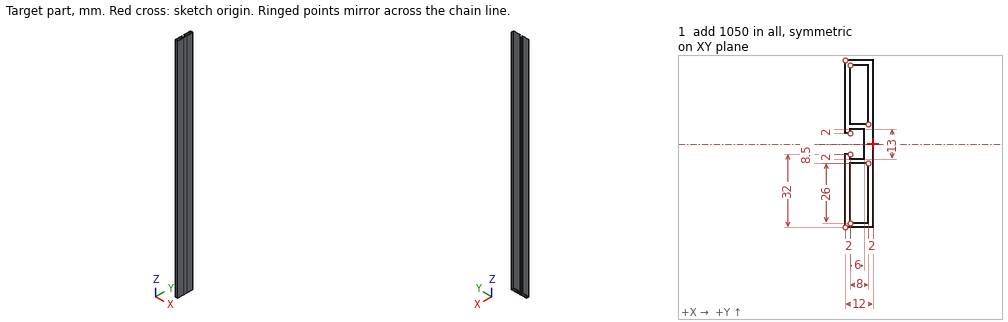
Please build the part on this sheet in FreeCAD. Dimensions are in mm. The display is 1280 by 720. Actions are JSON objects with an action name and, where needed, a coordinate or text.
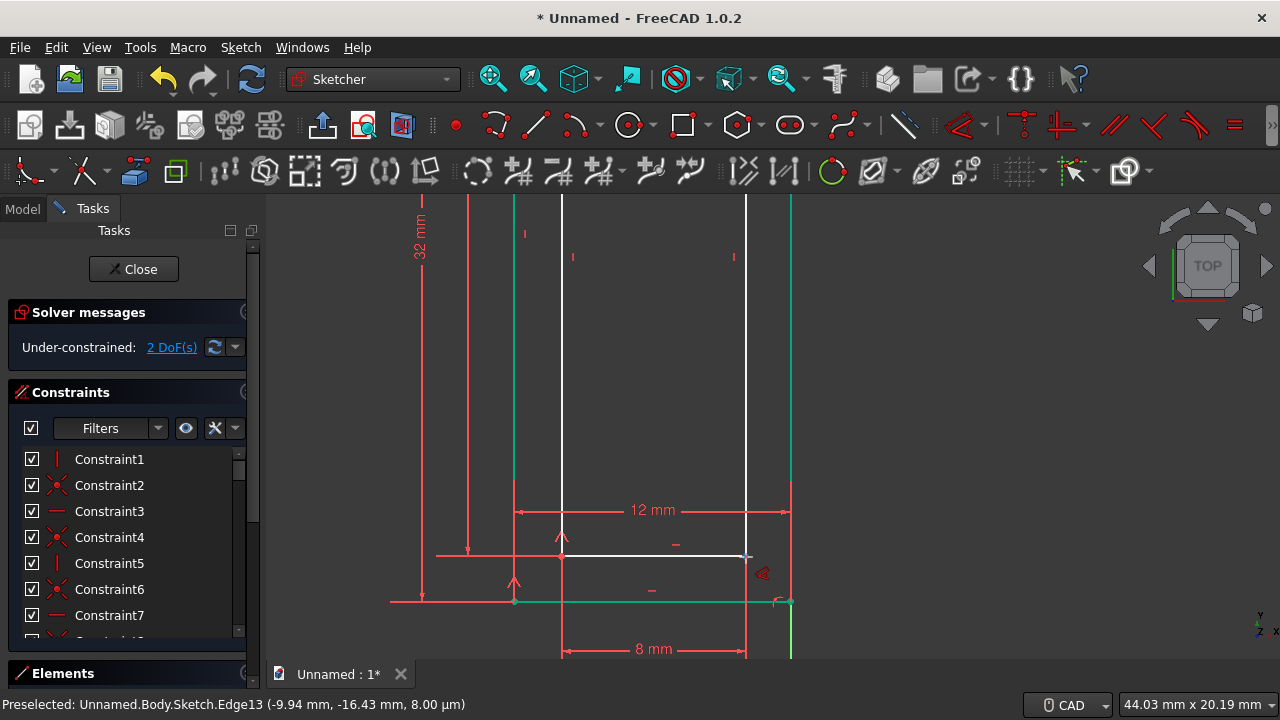
{"action": "left_click", "coordinate": [746, 556]}
{"action": "left_click", "coordinate": [768, 590]}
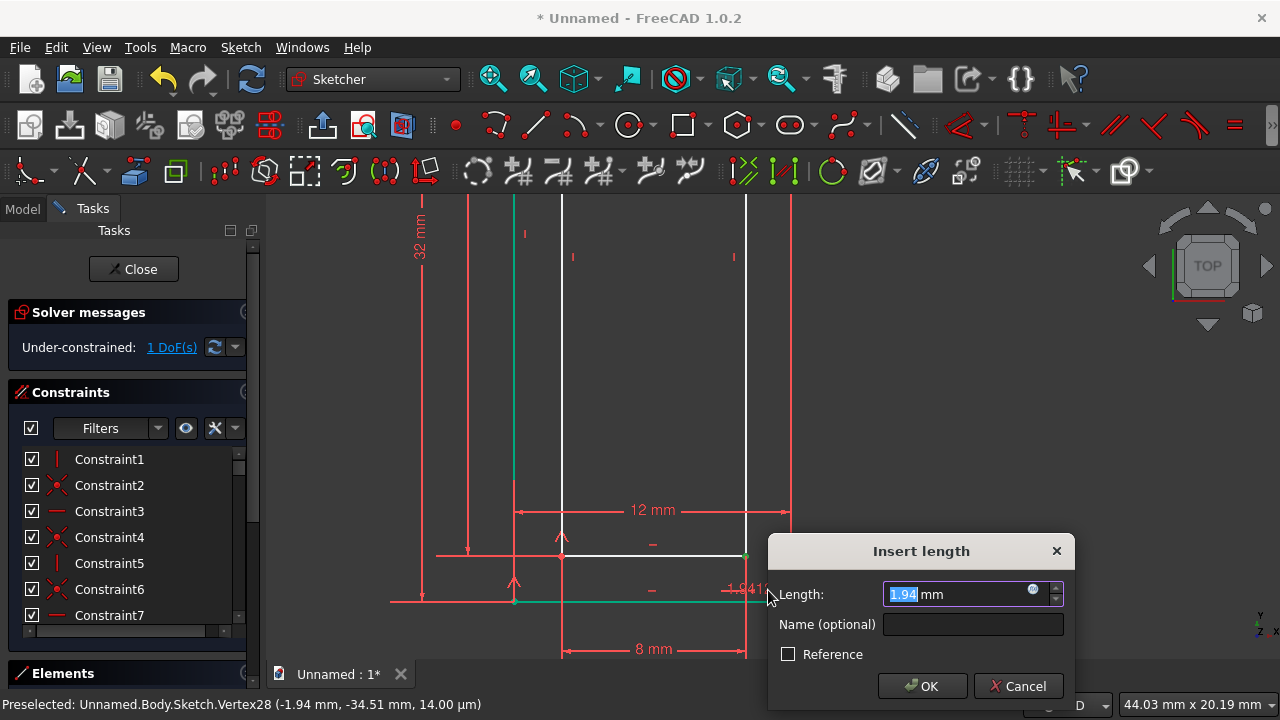
{"action": "type", "text": "2"}
{"action": "key", "text": "Return"}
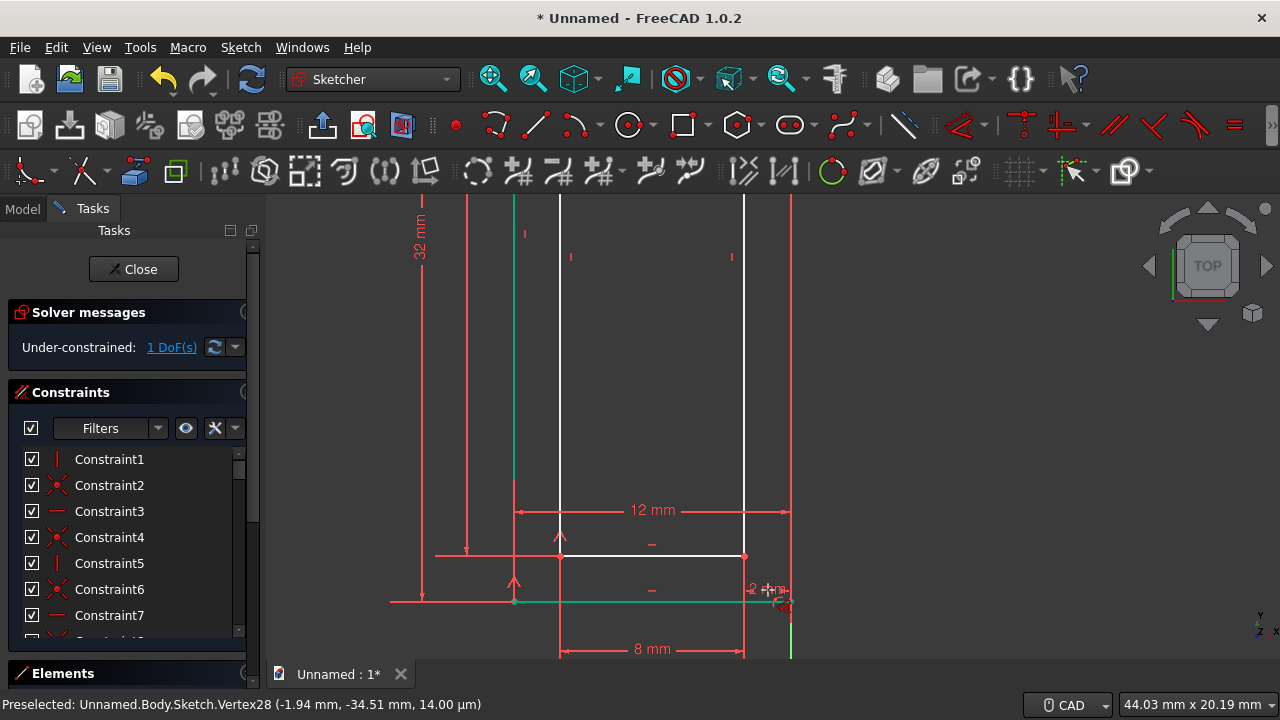
{"action": "scroll", "coordinate": [715, 558], "scroll_direction": "down", "scroll_amount": 9}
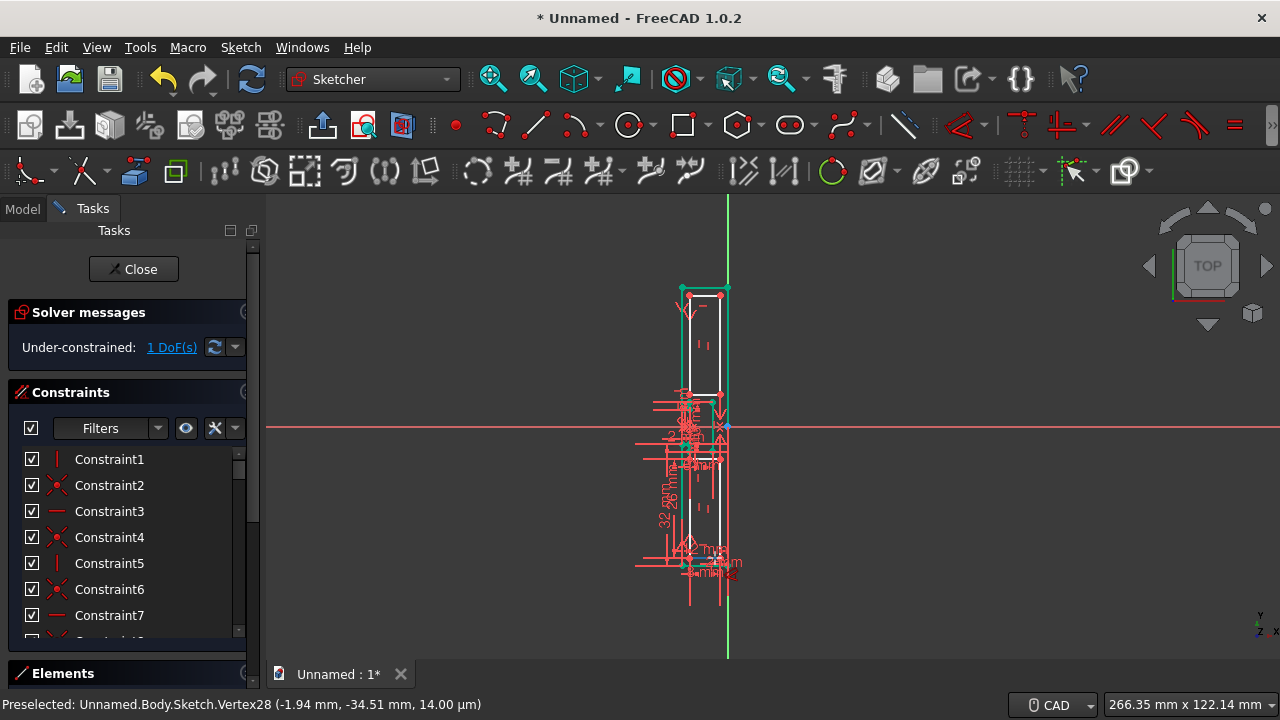
{"action": "scroll", "coordinate": [690, 459], "scroll_direction": "up", "scroll_amount": 3}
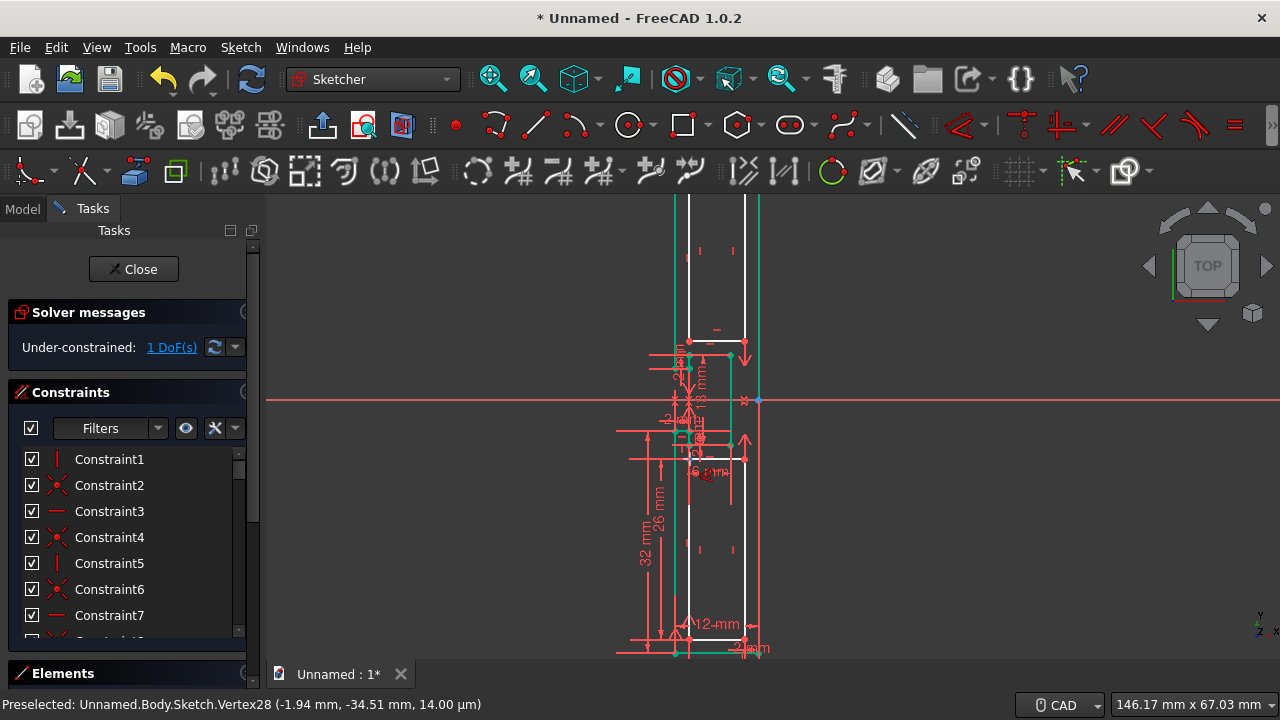
{"action": "left_click", "coordinate": [689, 459]}
{"action": "left_click", "coordinate": [793, 430]}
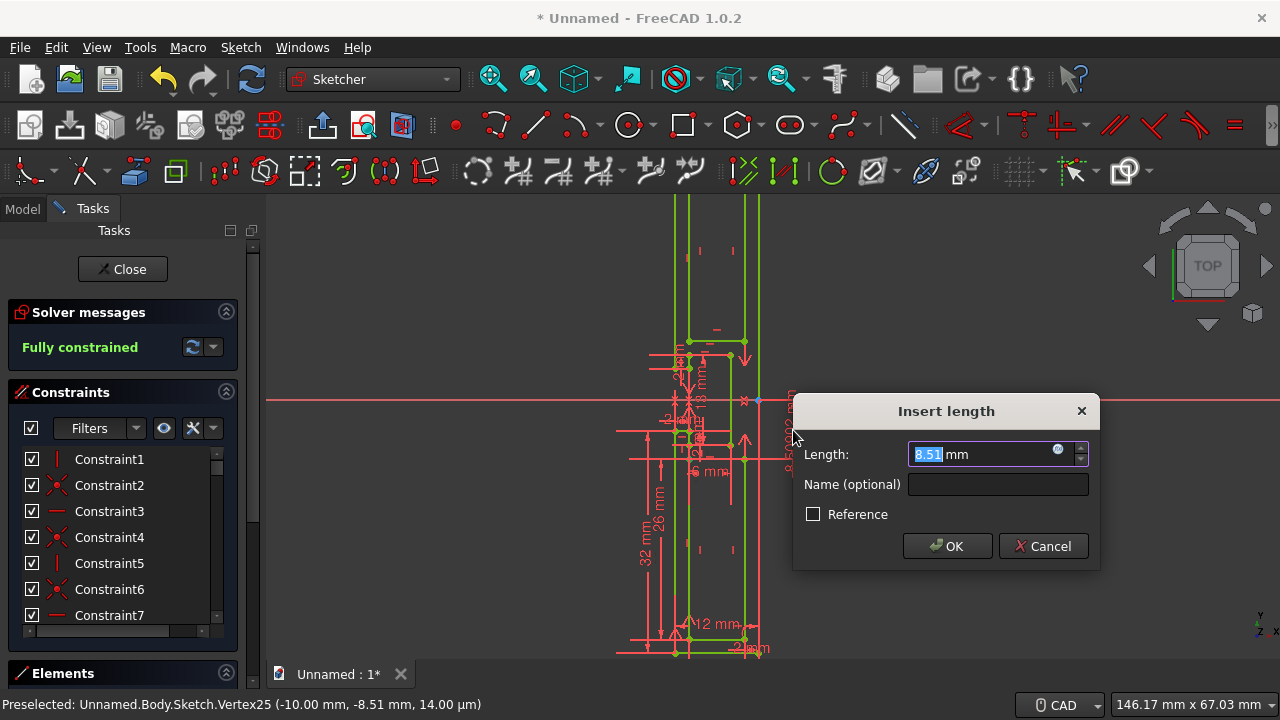
{"action": "type", "text": "8.5"}
{"action": "key", "text": "Return"}
{"action": "key", "text": "Escape"}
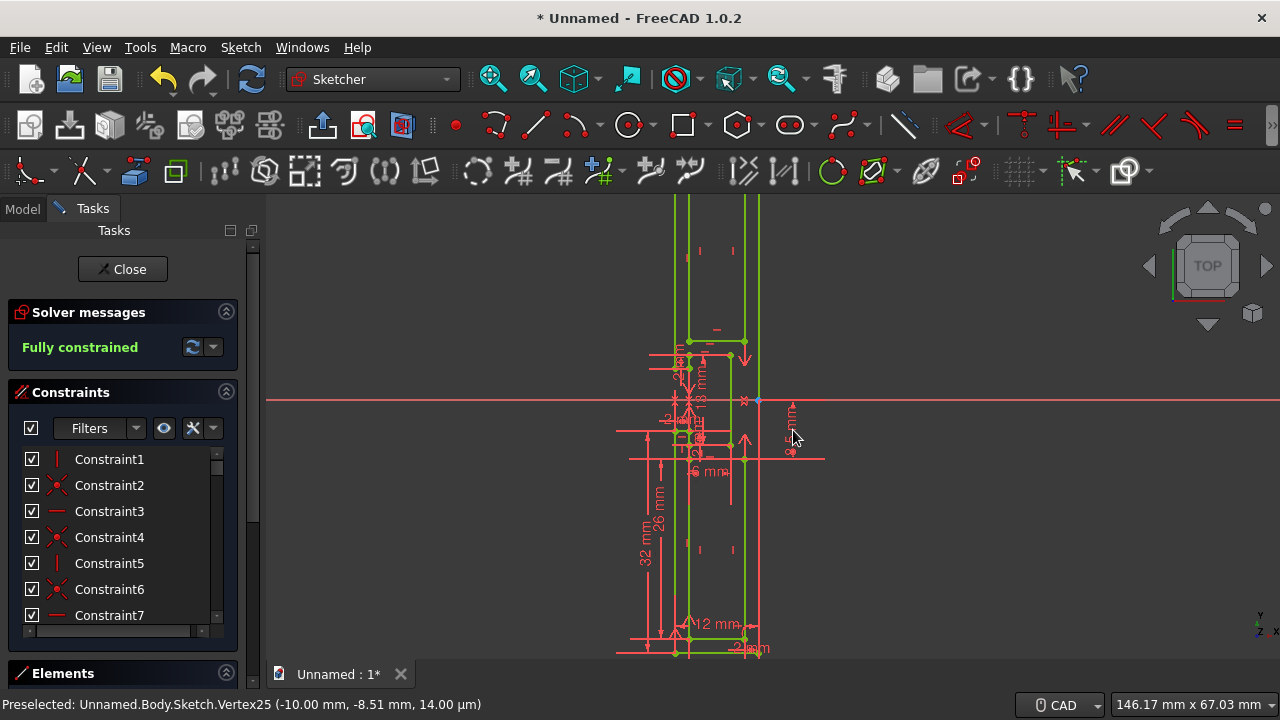
{"action": "left_click", "coordinate": [123, 269]}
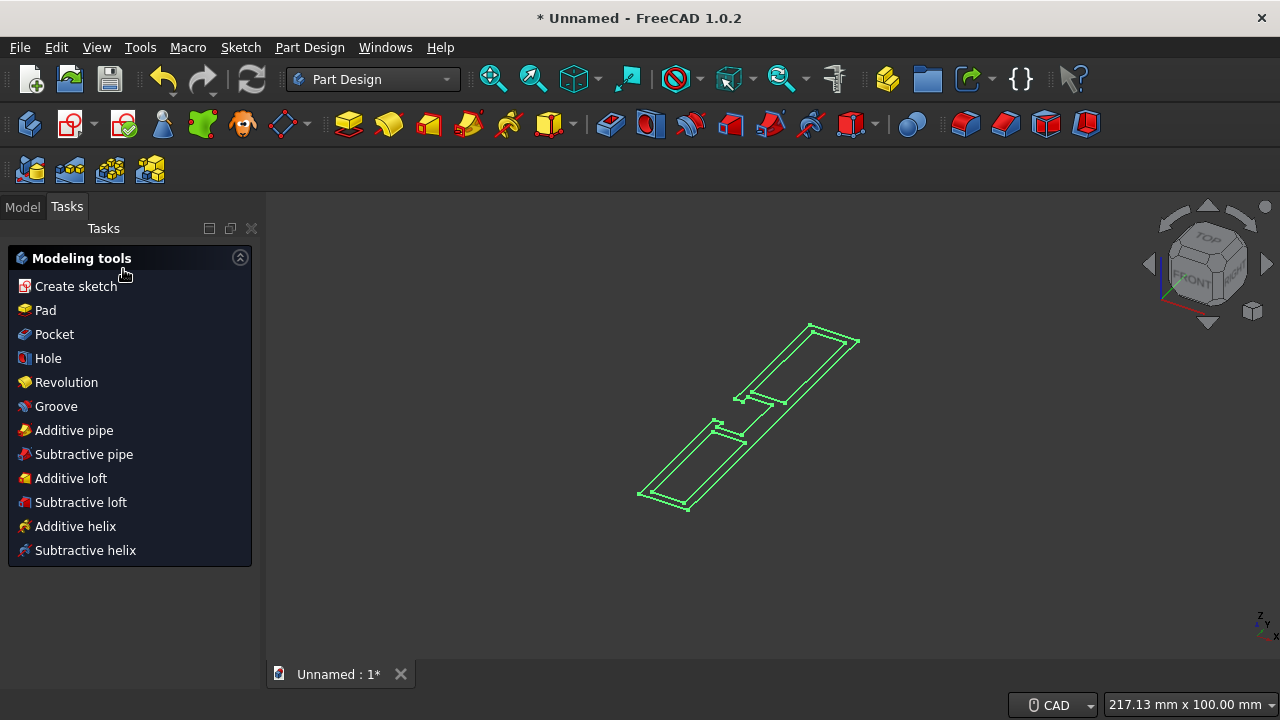
{"action": "left_click", "coordinate": [350, 124]}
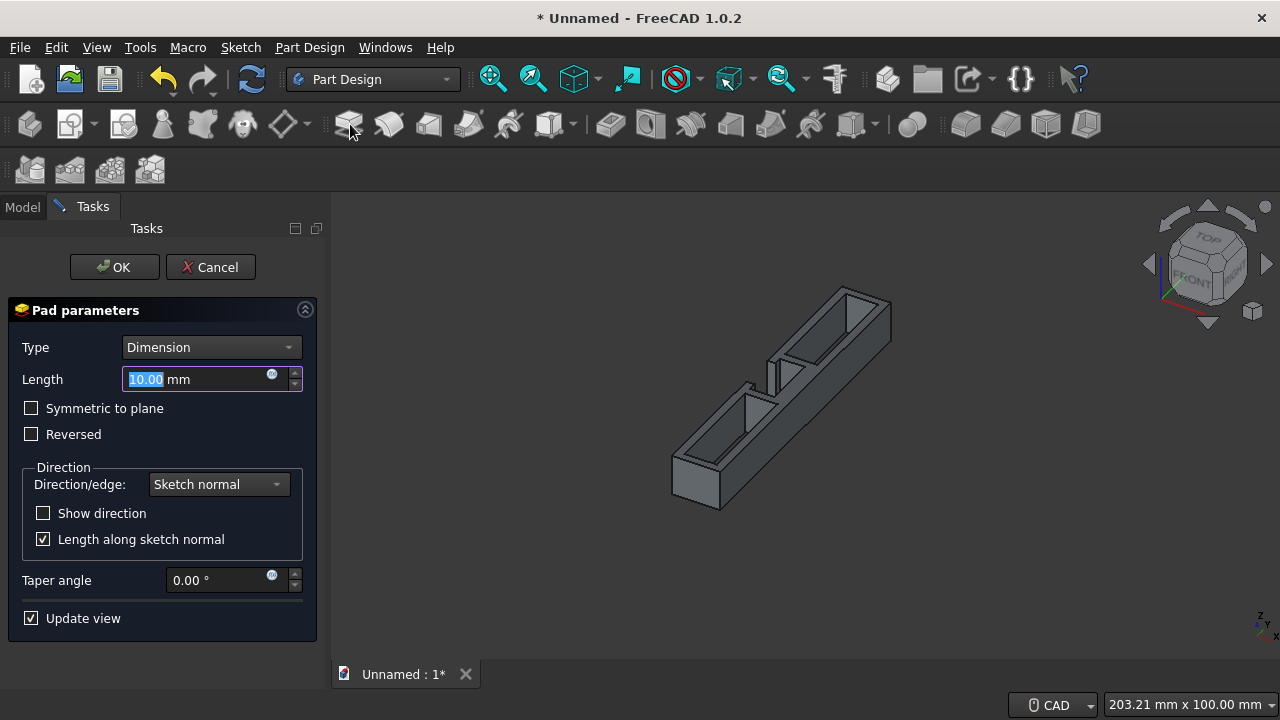
{"action": "type", "text": "1050"}
{"action": "key", "text": "Tab"}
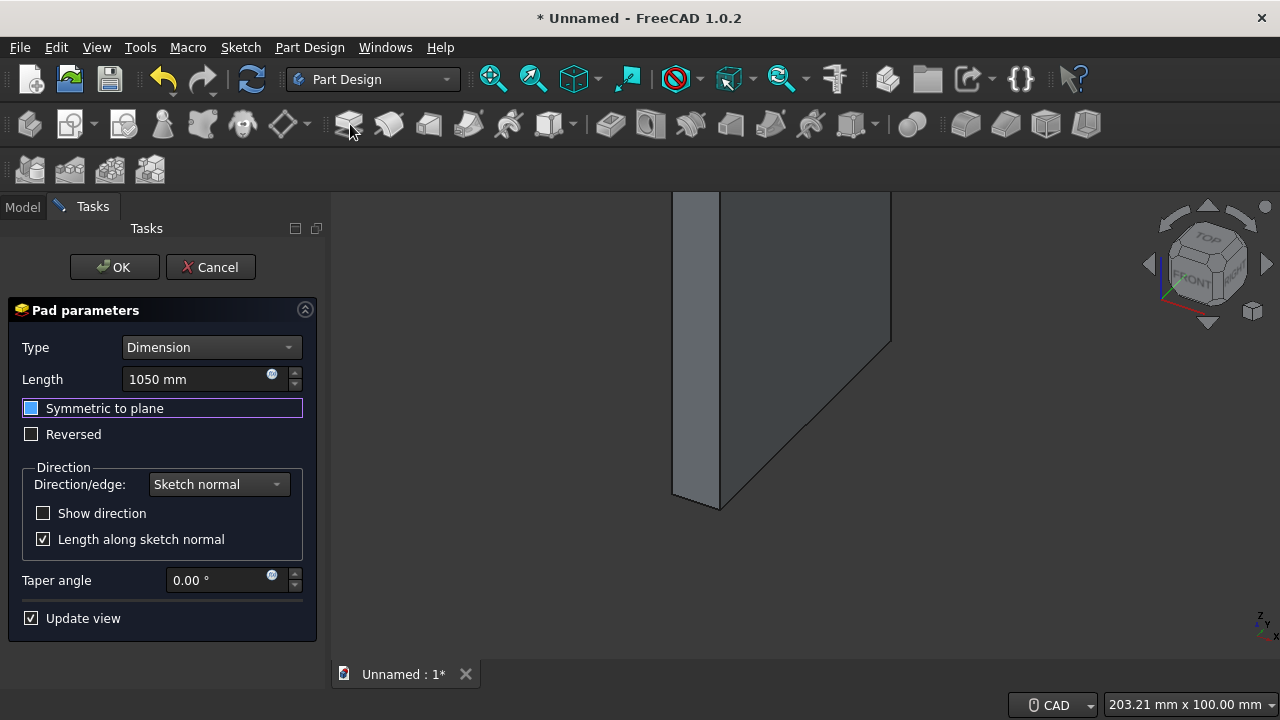
{"action": "left_click", "coordinate": [30, 408]}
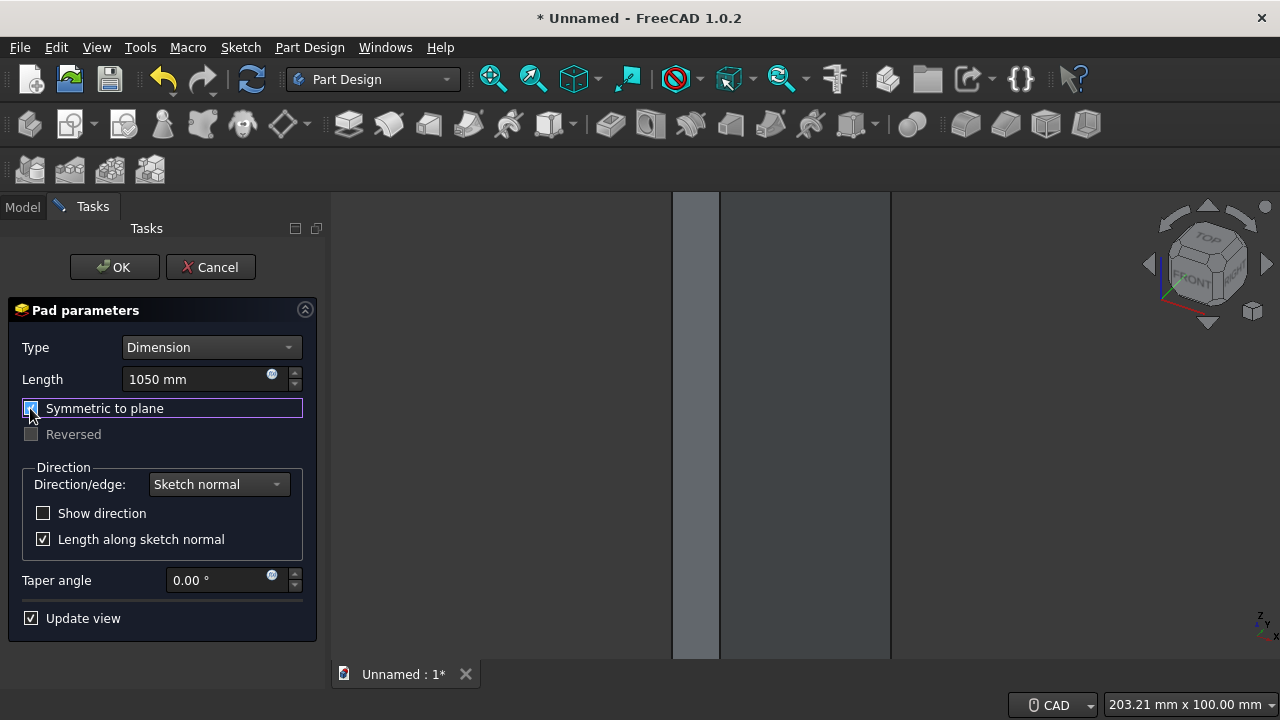
{"action": "left_click", "coordinate": [115, 267]}